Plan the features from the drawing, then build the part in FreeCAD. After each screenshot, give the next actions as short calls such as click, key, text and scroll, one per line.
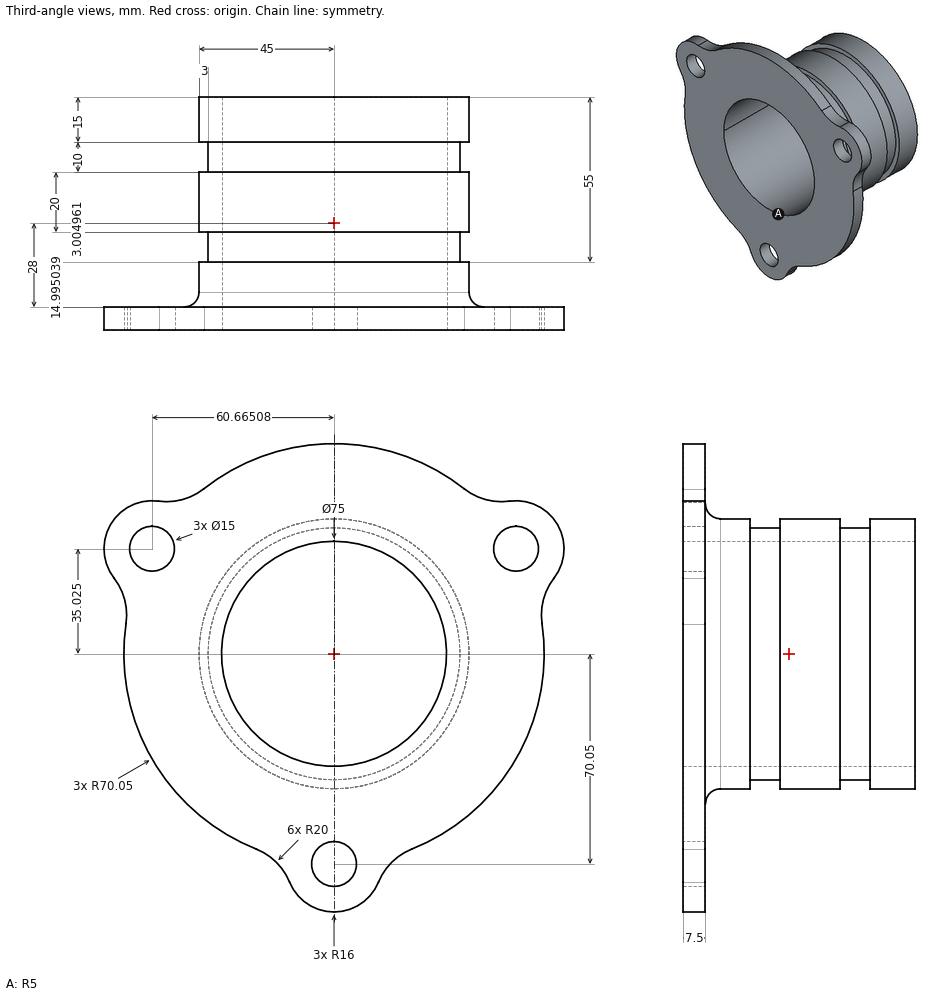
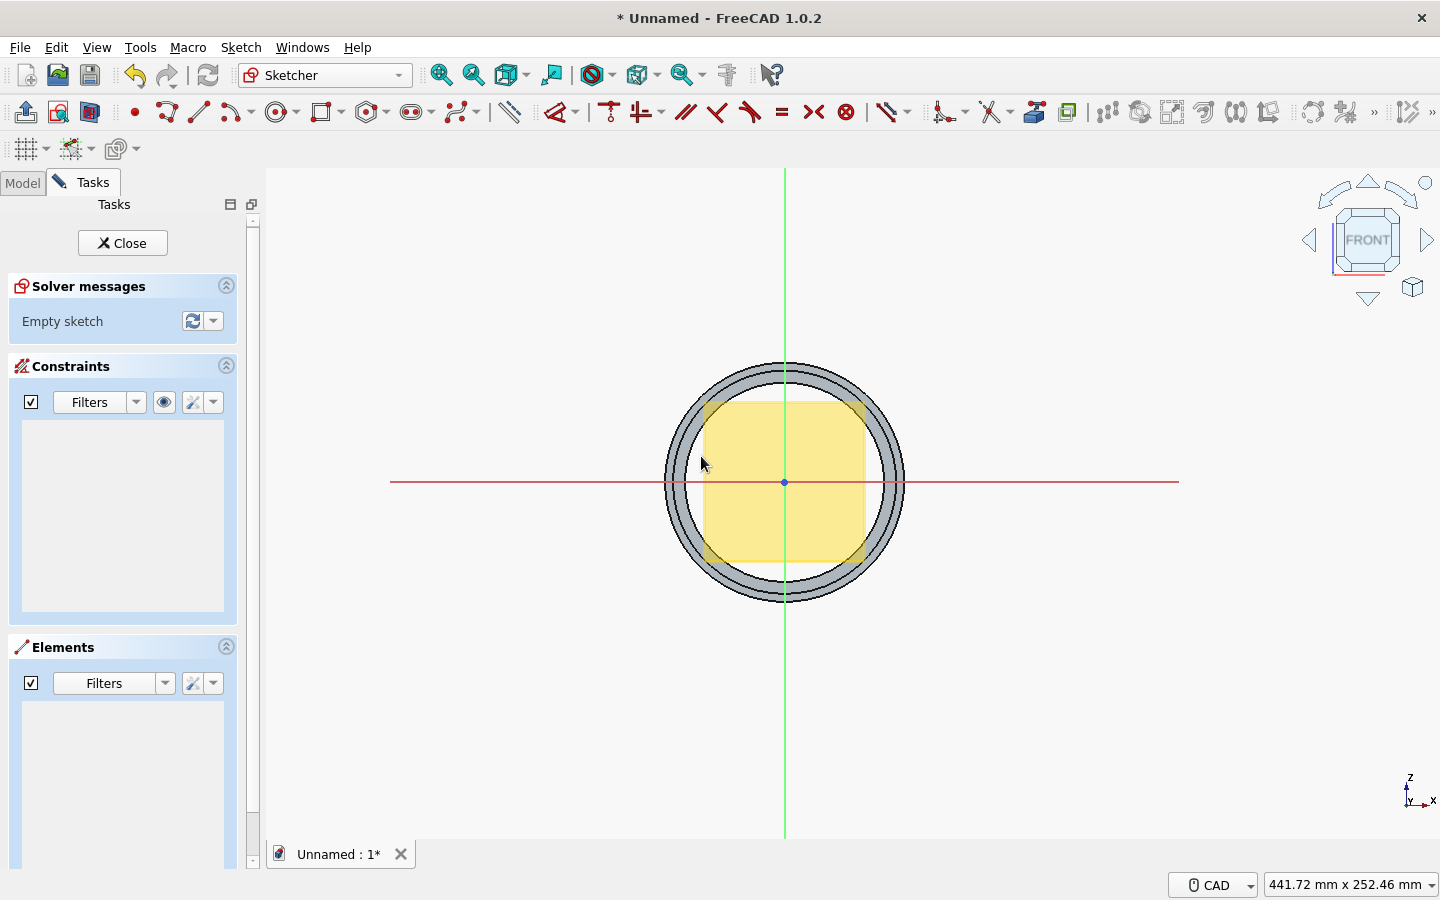
click(254, 112)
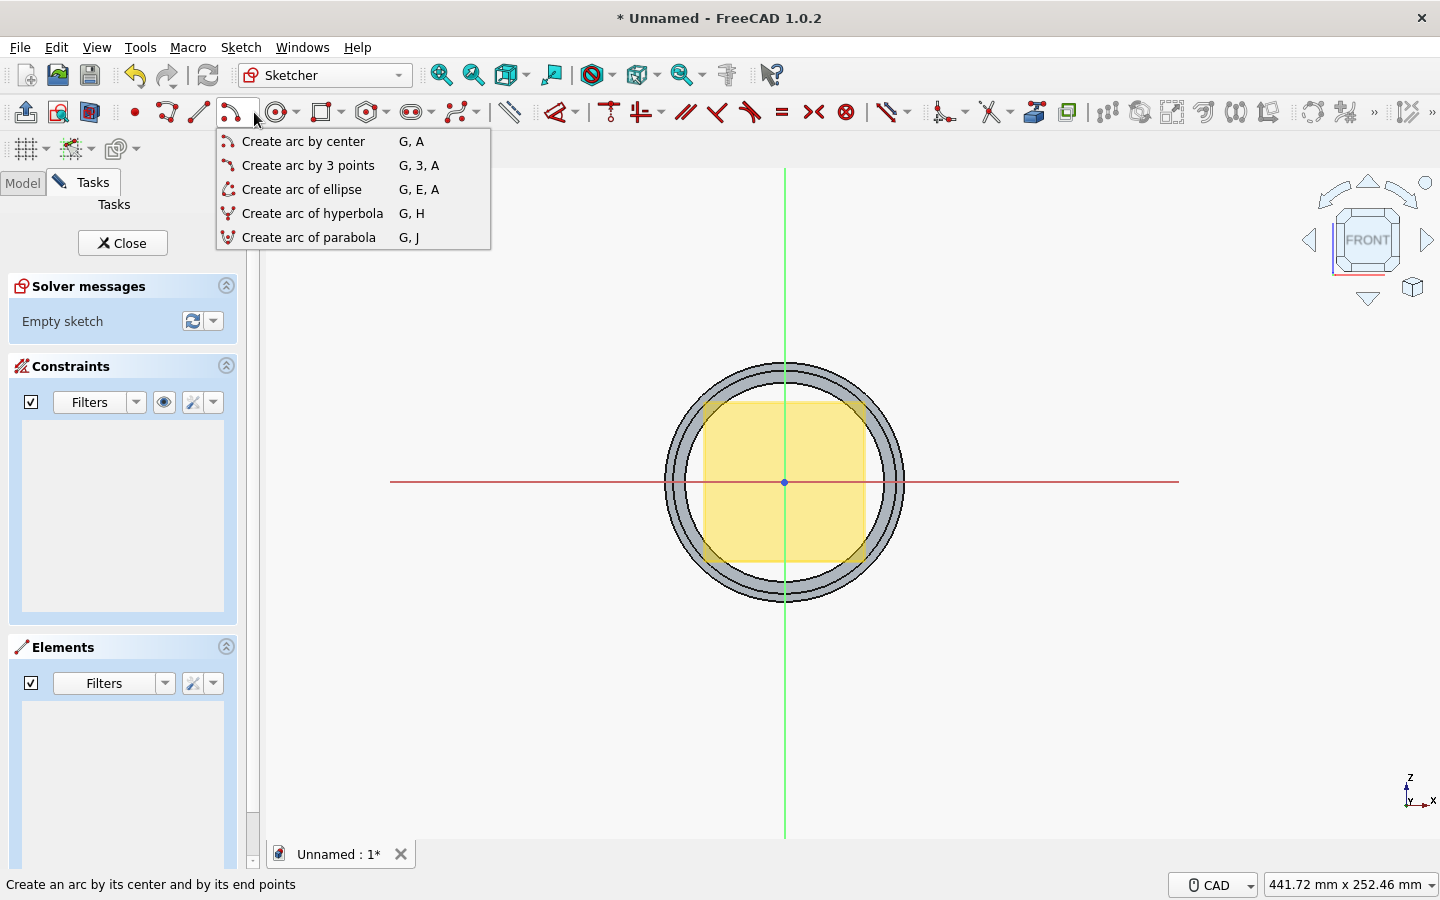
click(354, 165)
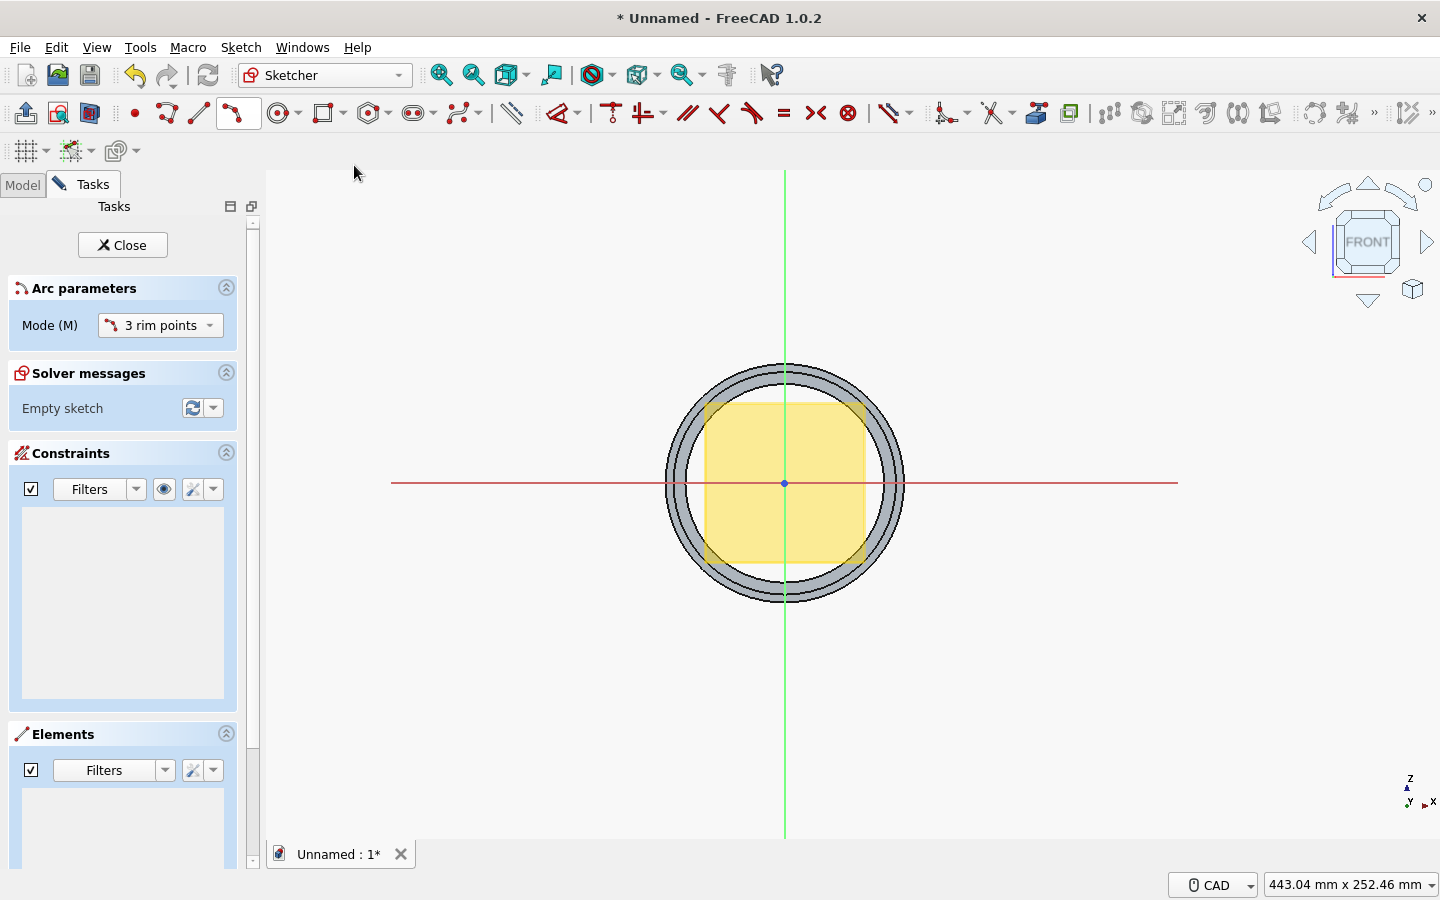
click(601, 457)
click(591, 416)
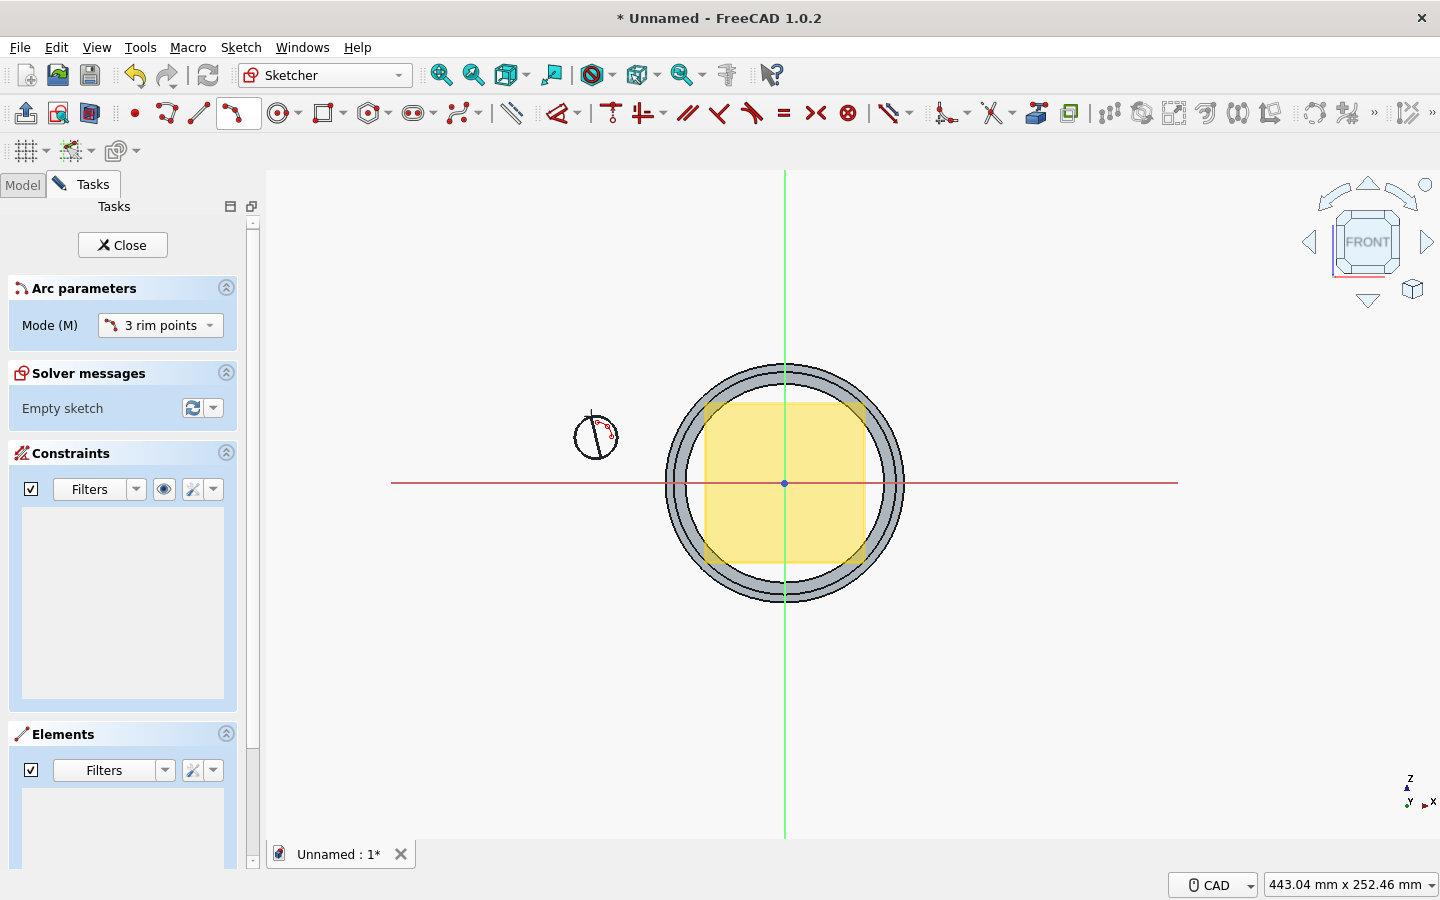
scroll(600, 435, up, 7)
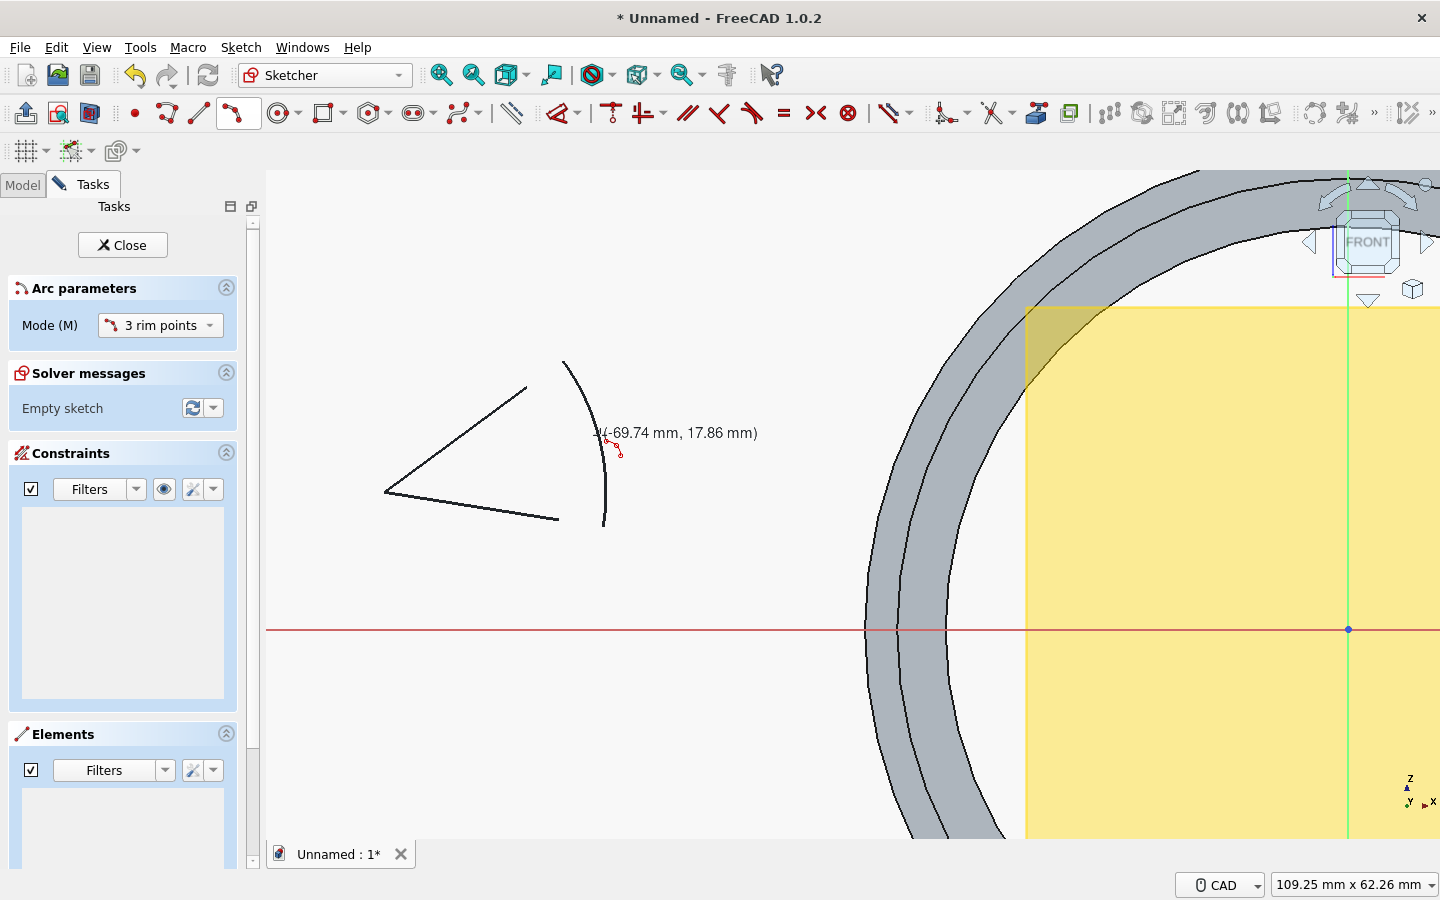
click(599, 436)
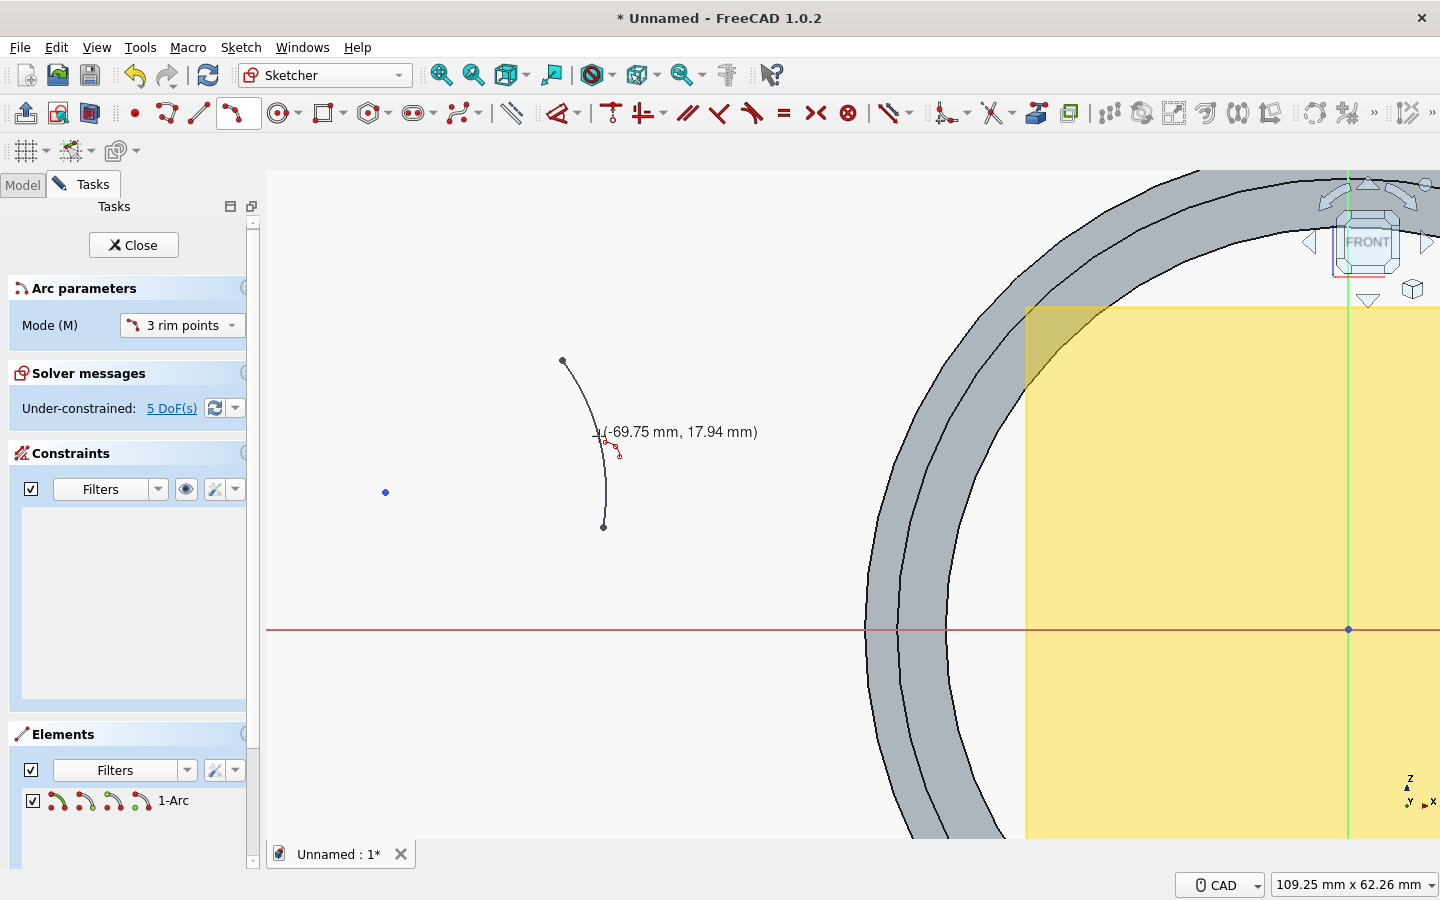
scroll(600, 435, down, 7)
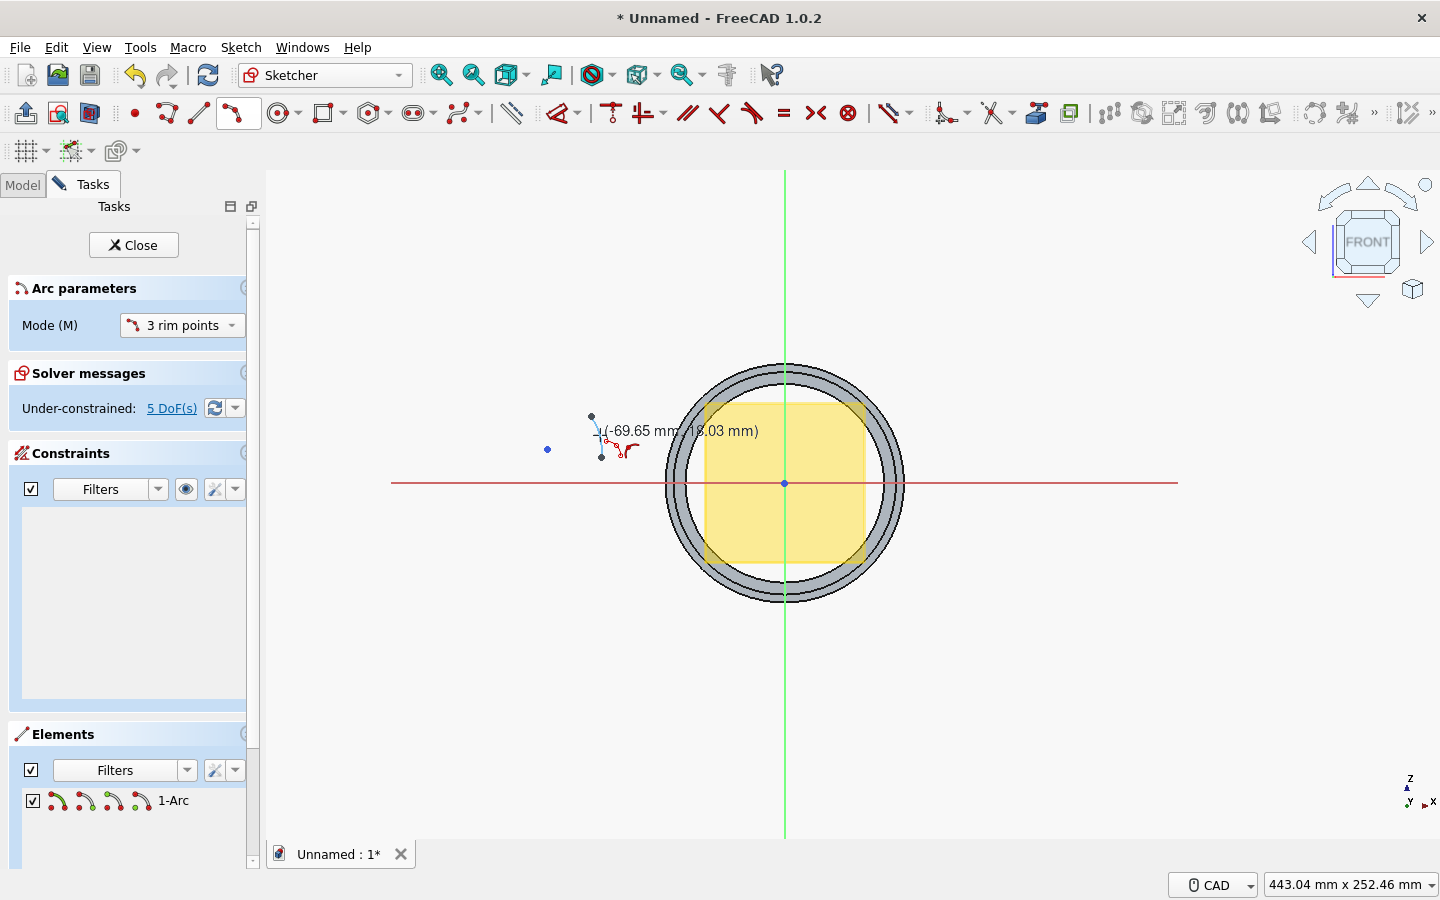
click(591, 417)
click(630, 349)
click(587, 369)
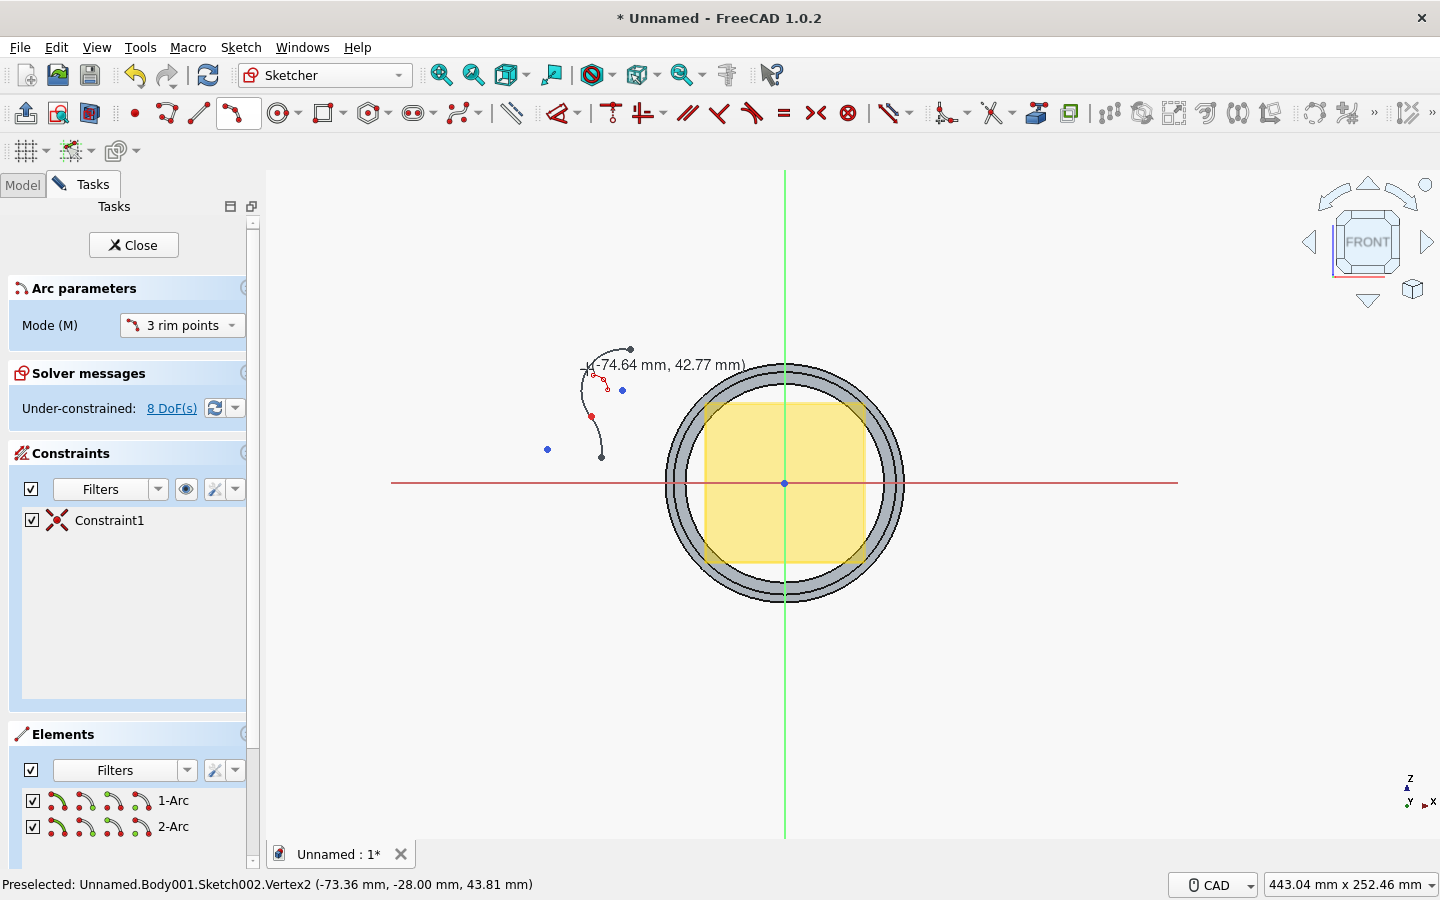
click(630, 350)
click(670, 338)